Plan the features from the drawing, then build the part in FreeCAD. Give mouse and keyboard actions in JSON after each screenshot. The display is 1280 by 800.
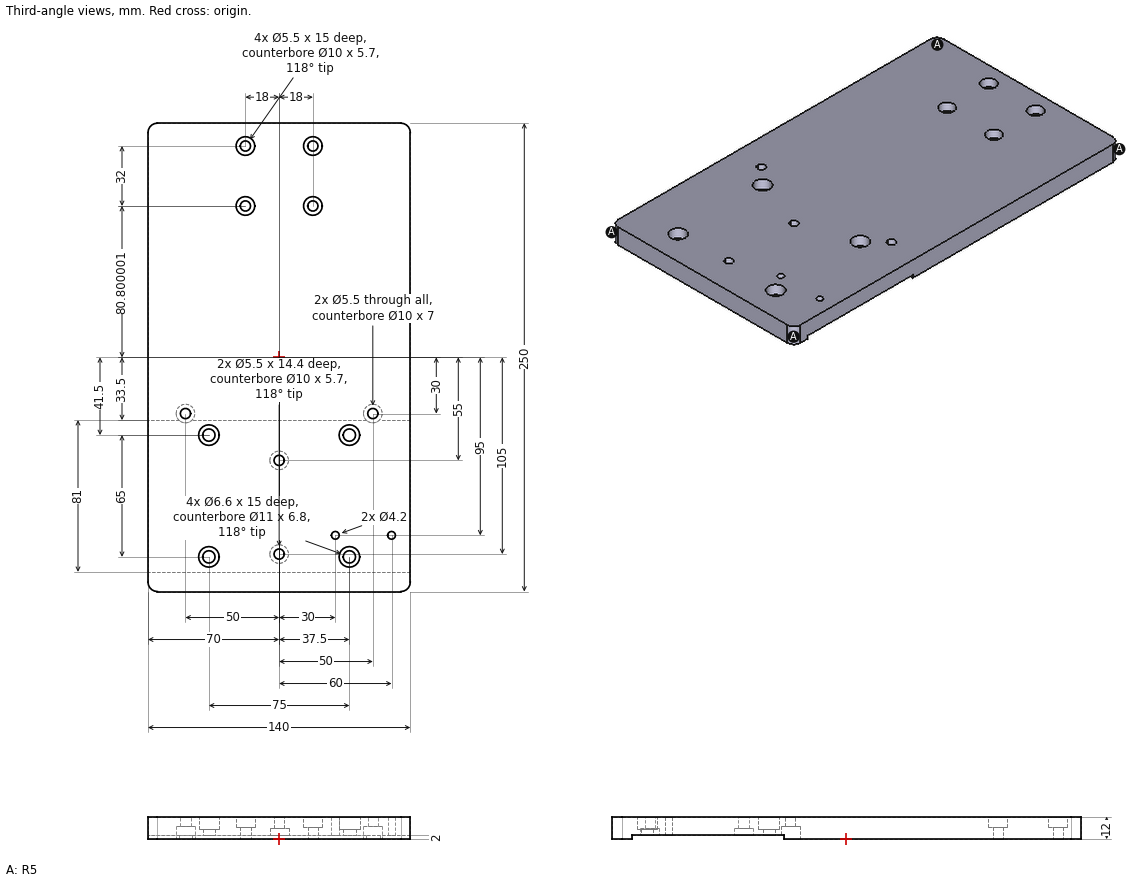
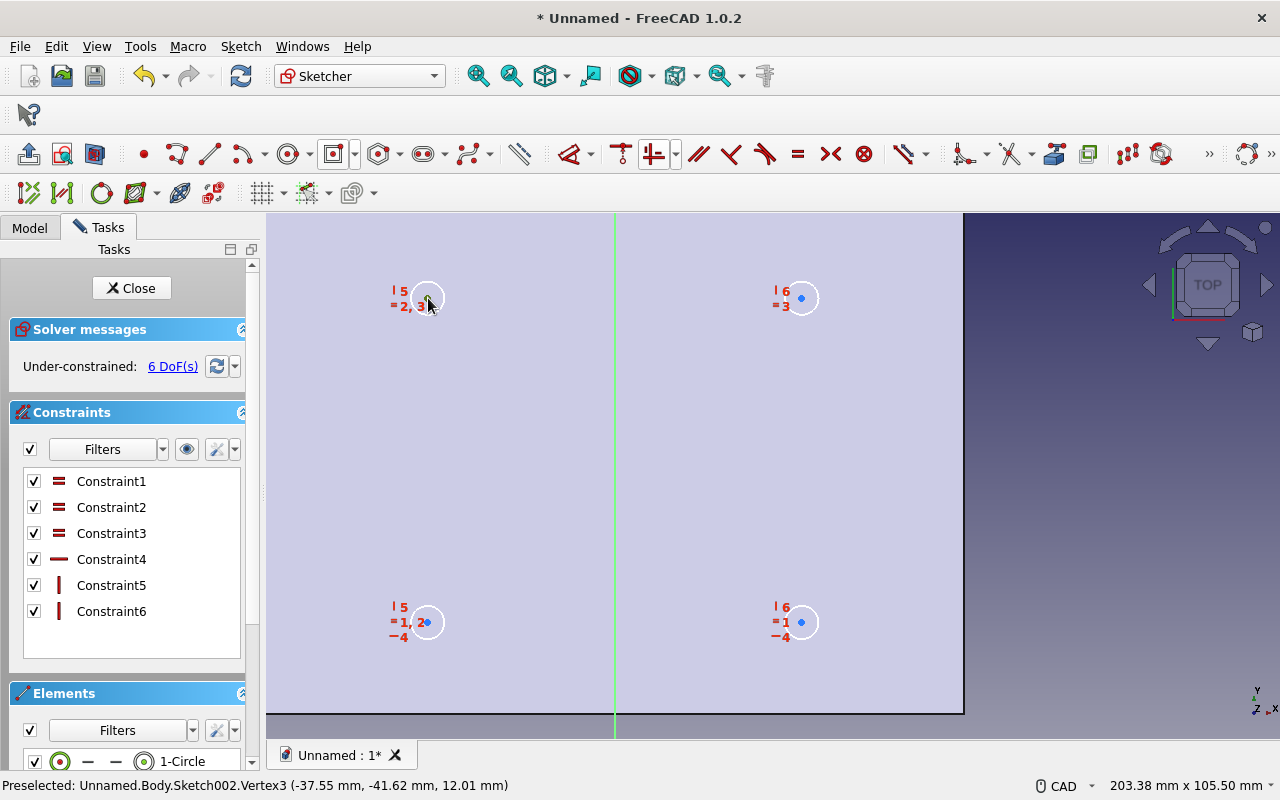
{"action": "left_click", "coordinate": [802, 298]}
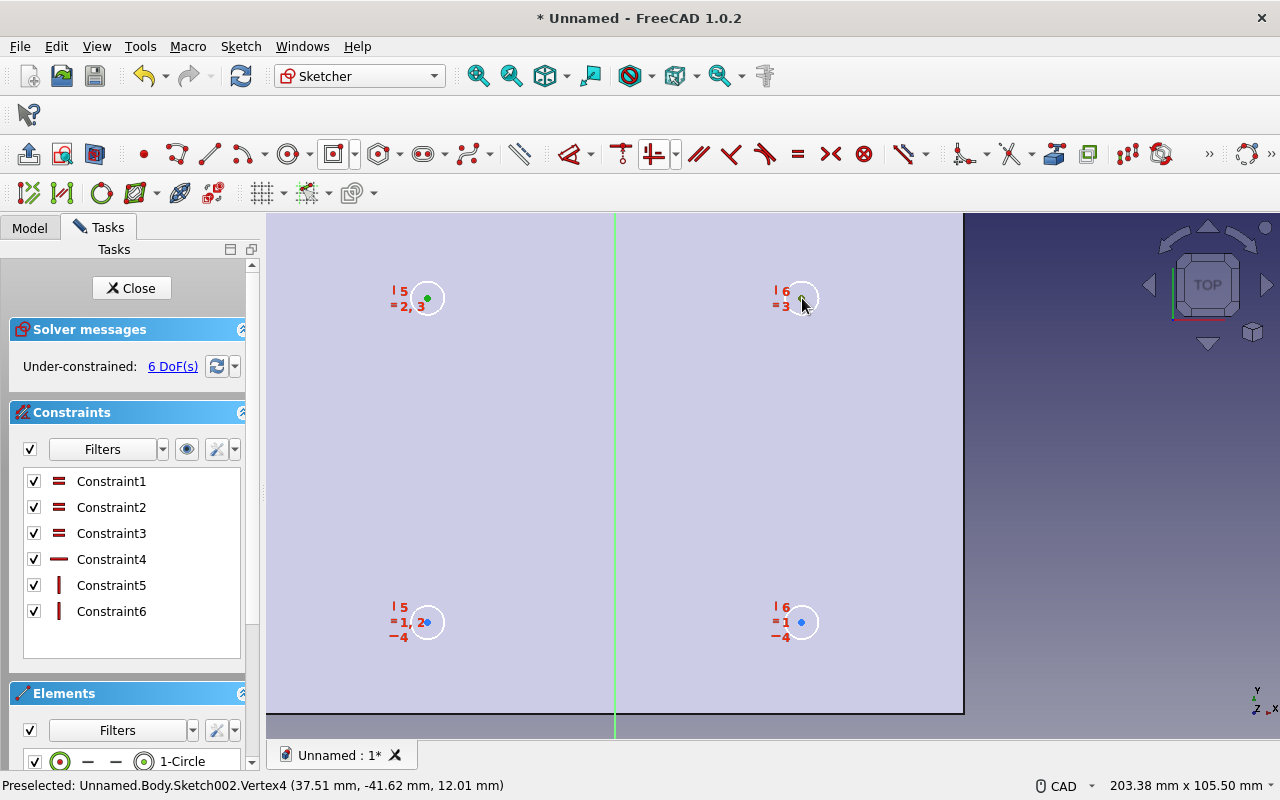
{"action": "left_click", "coordinate": [676, 154]}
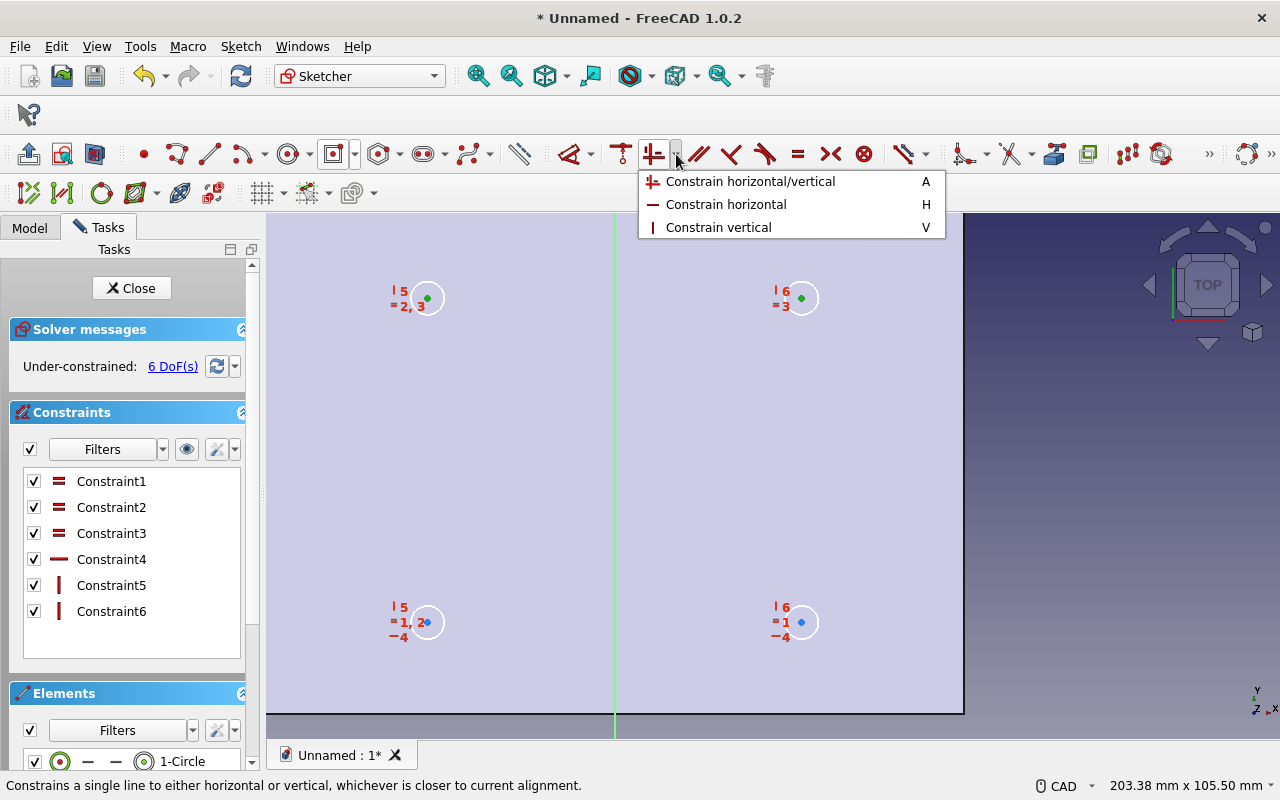
{"action": "left_click", "coordinate": [792, 204]}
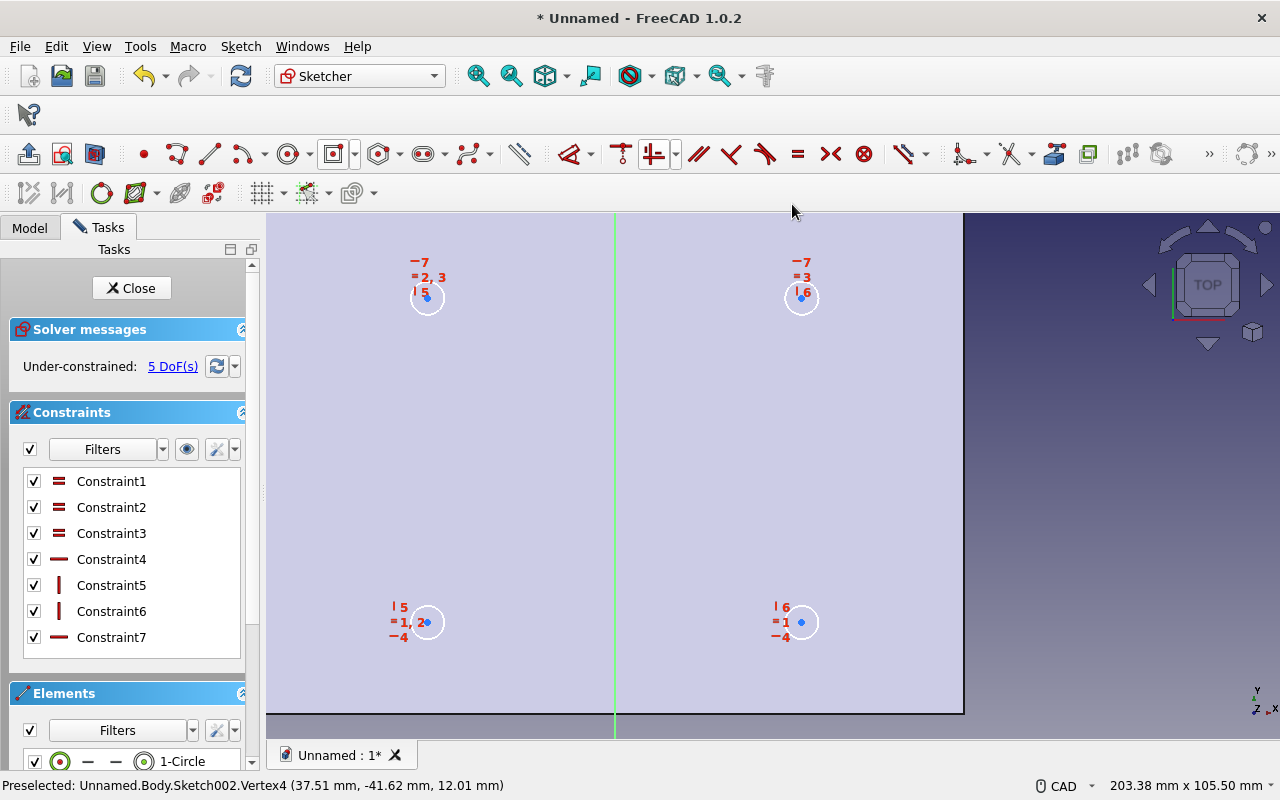
{"action": "left_click", "coordinate": [814, 611]}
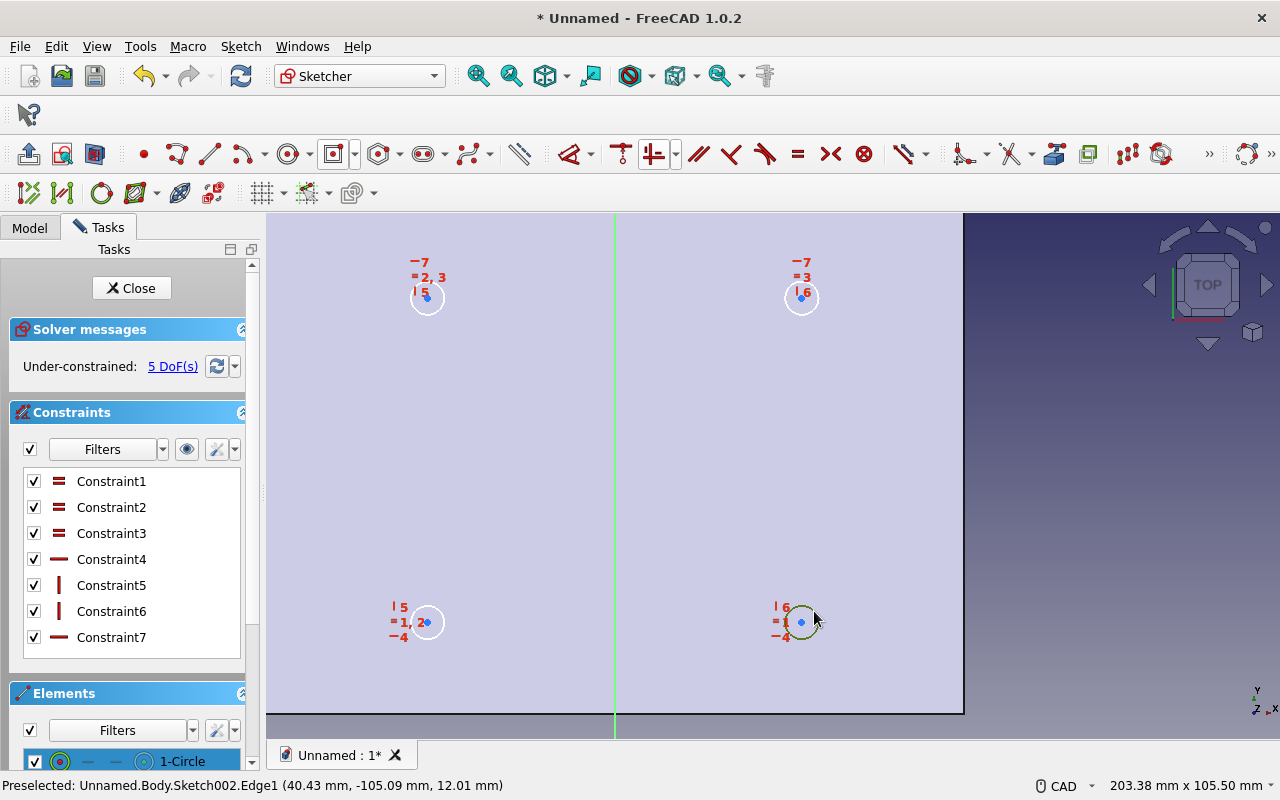
{"action": "left_click", "coordinate": [590, 154]}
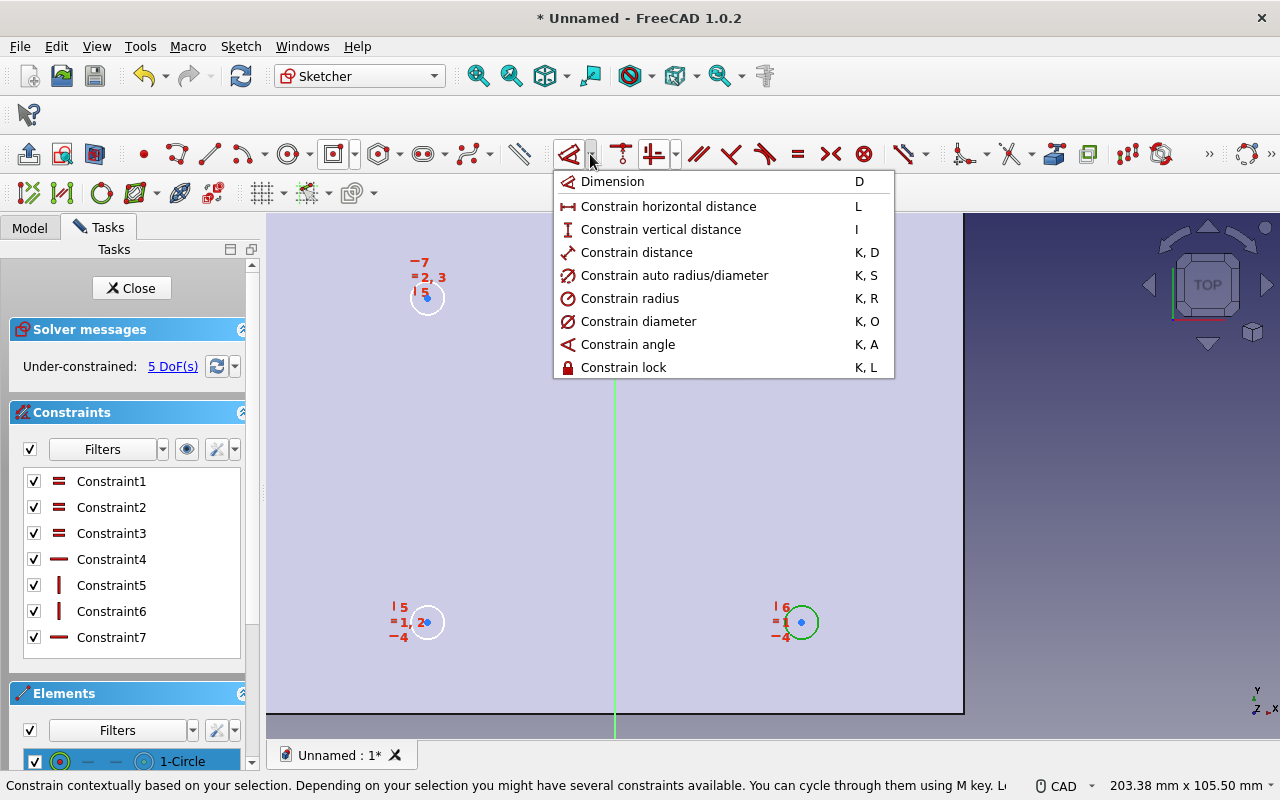
{"action": "left_click", "coordinate": [724, 322]}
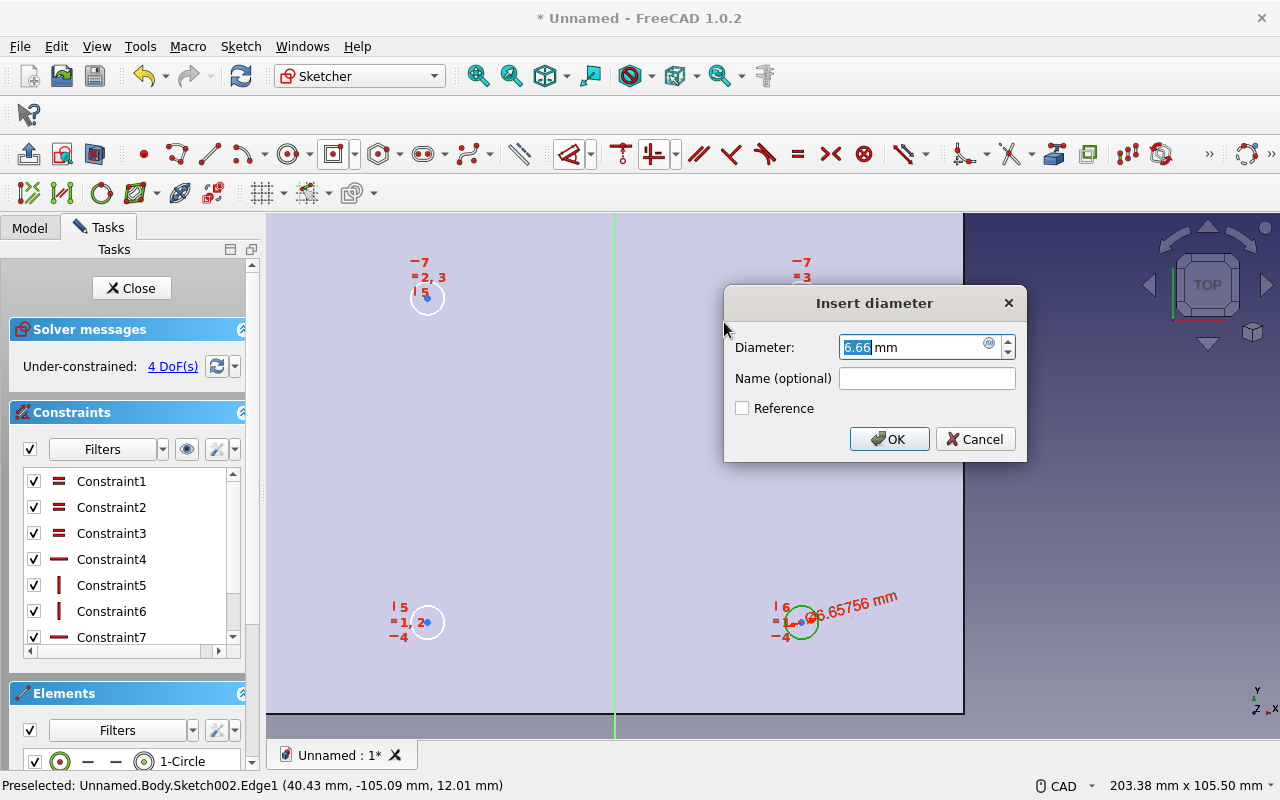
{"action": "type", "text": "6.6"}
{"action": "key", "text": "Return"}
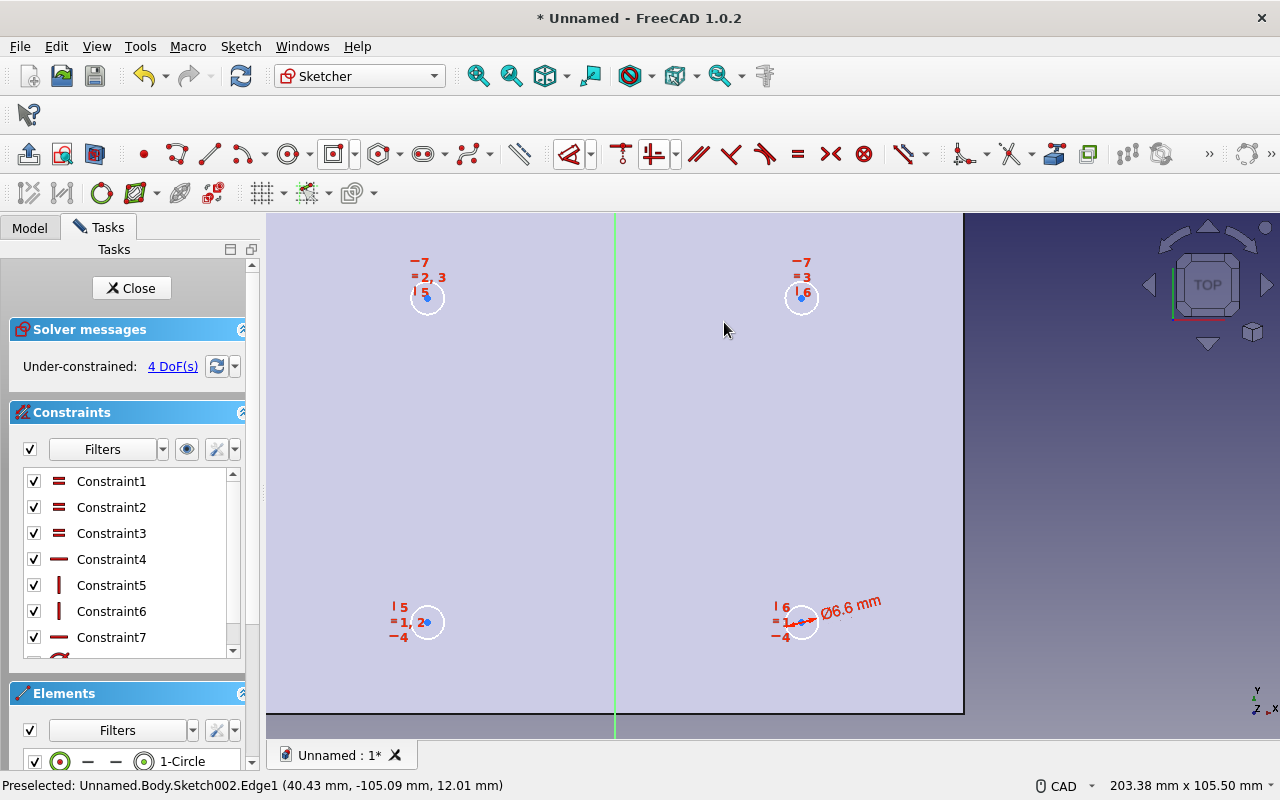
{"action": "left_click", "coordinate": [802, 623]}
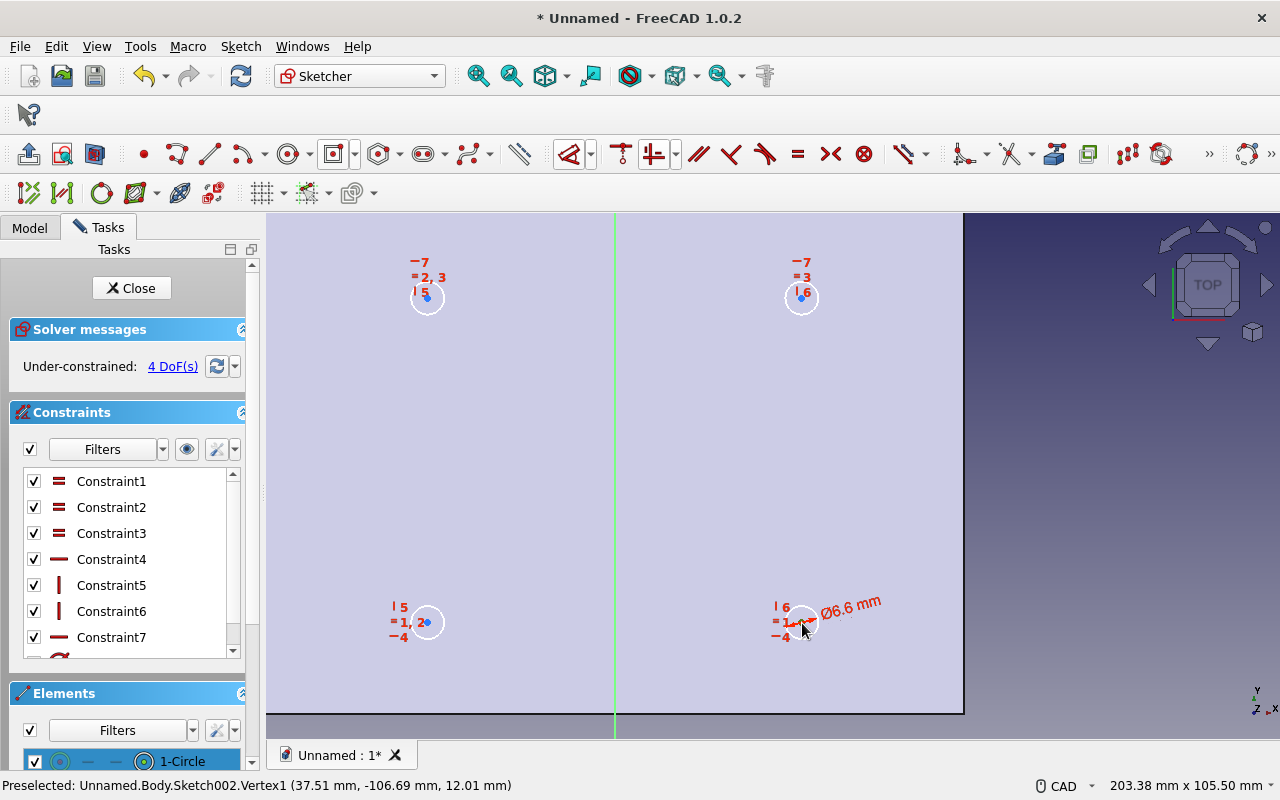
{"action": "left_click", "coordinate": [428, 623]}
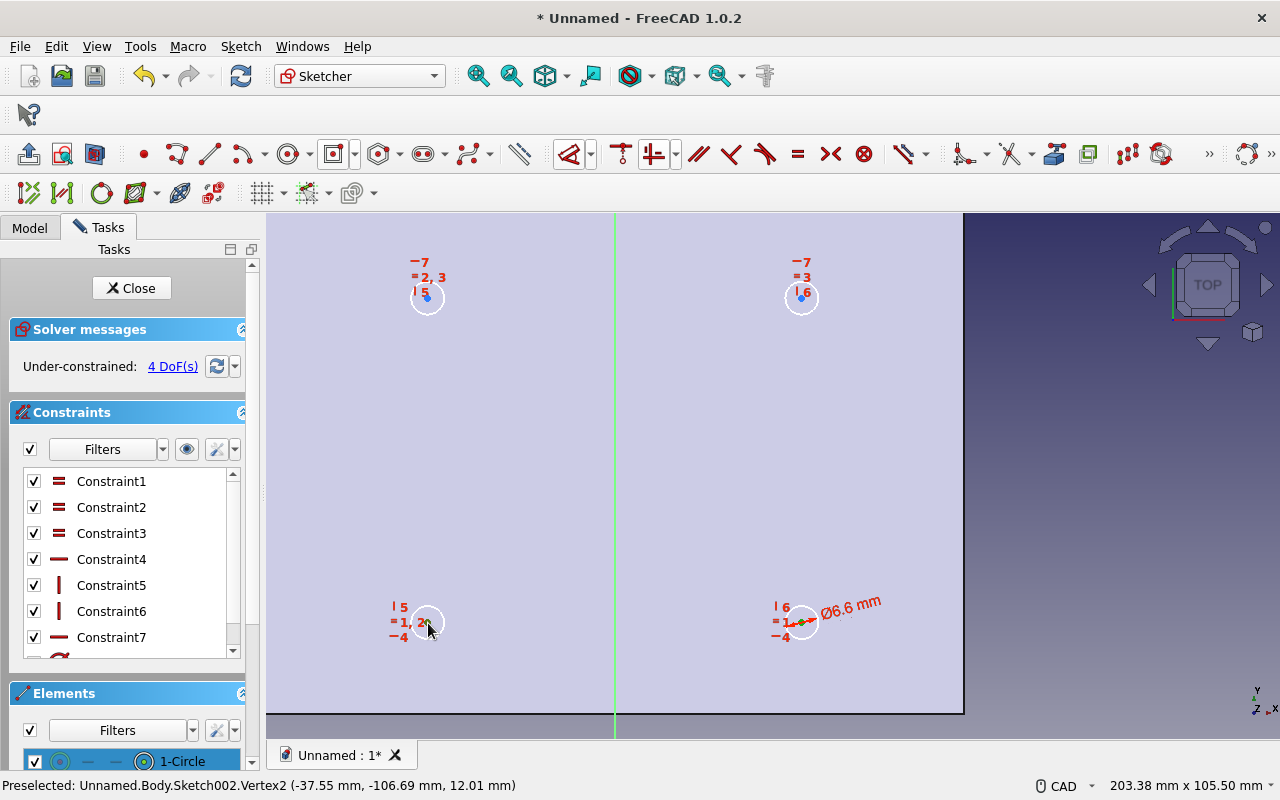
{"action": "left_click", "coordinate": [590, 154]}